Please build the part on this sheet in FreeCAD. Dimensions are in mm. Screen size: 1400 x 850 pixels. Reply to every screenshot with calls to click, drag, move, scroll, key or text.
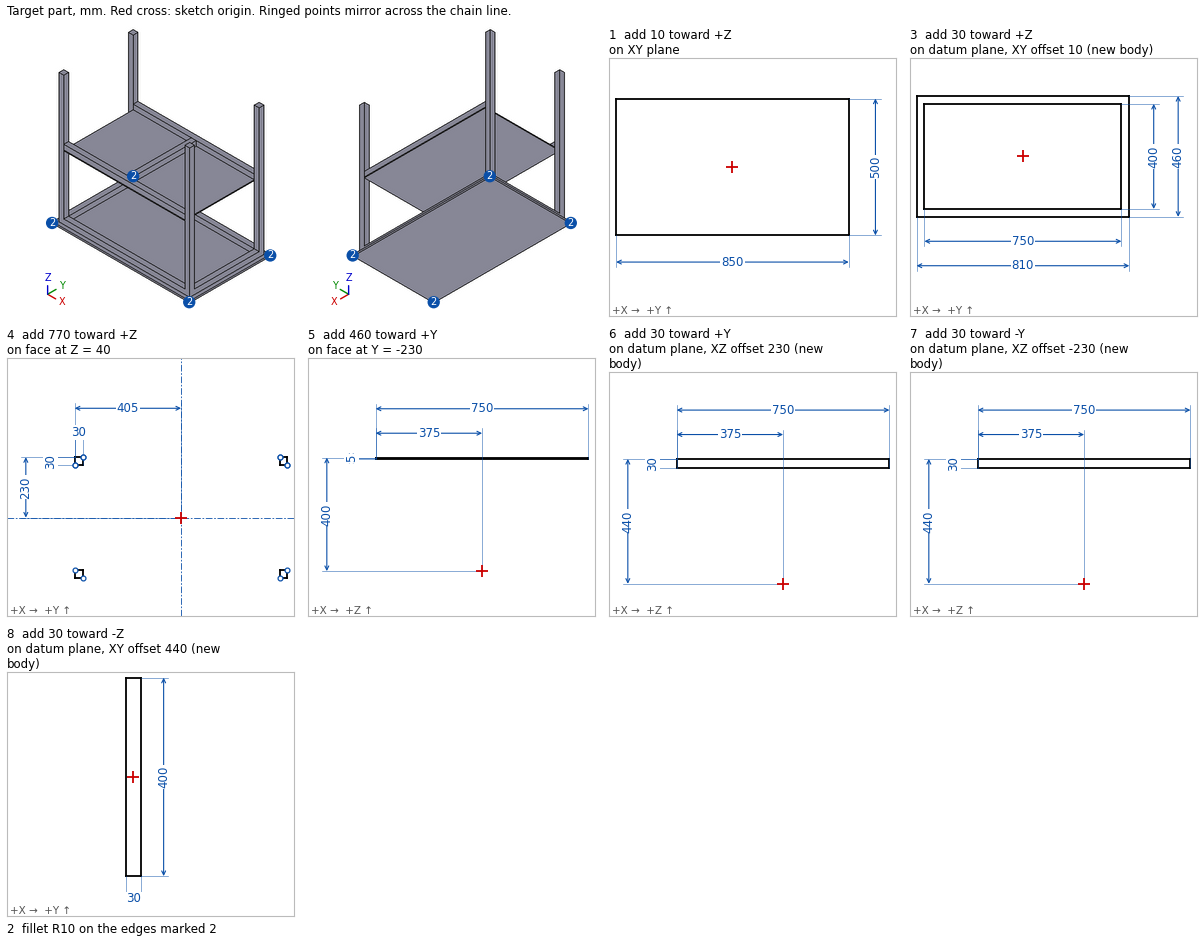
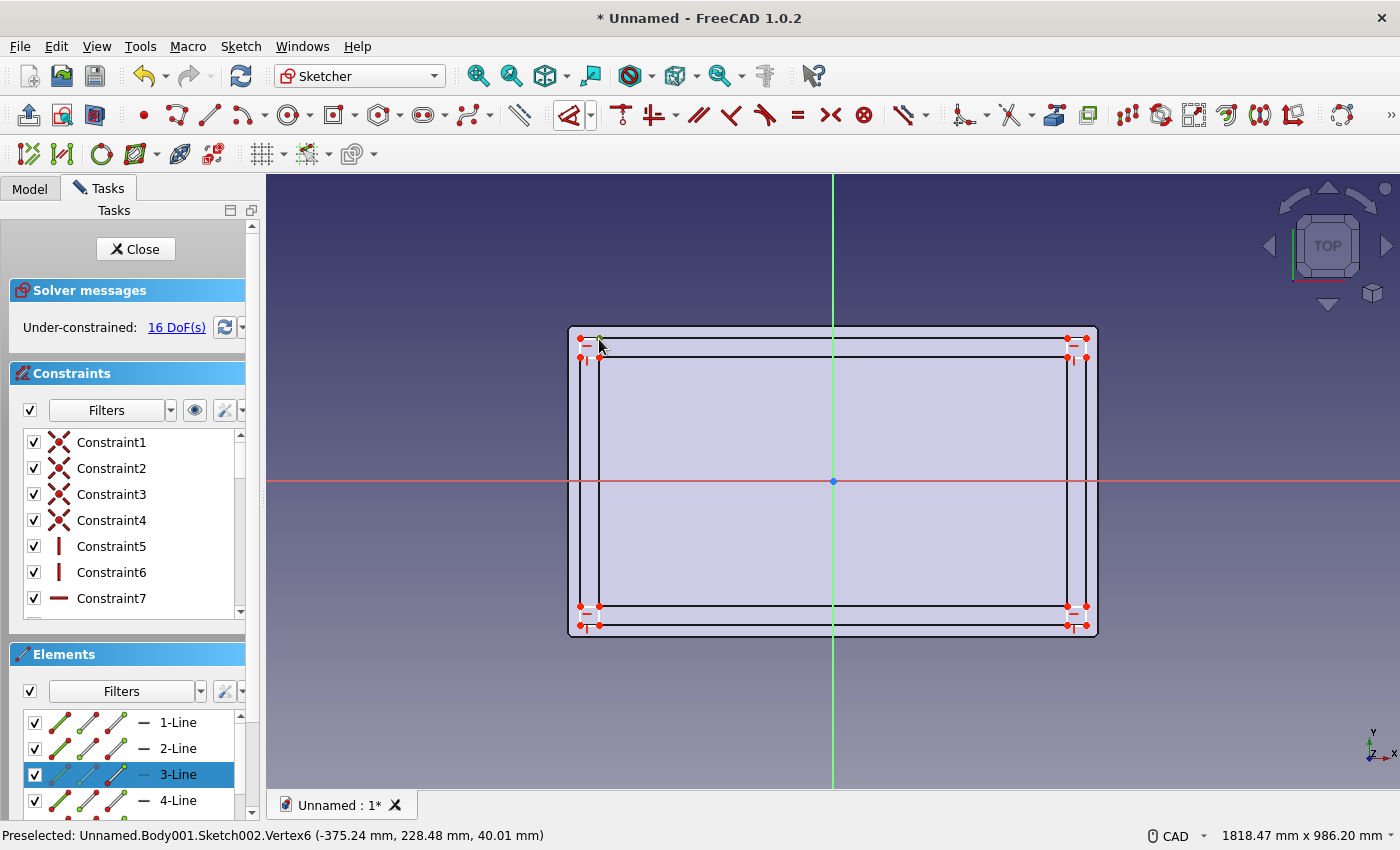
click(1067, 339)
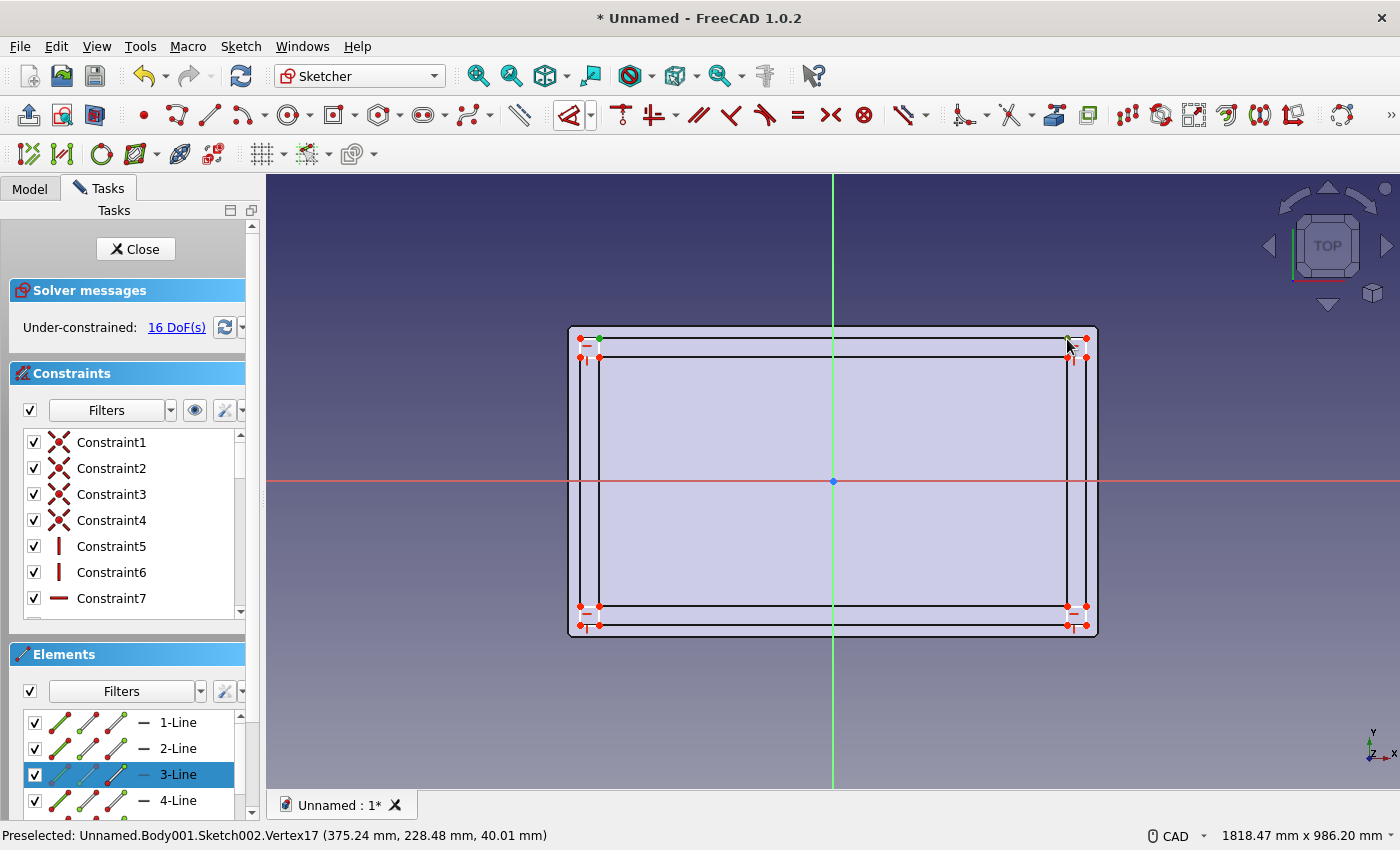
click(833, 721)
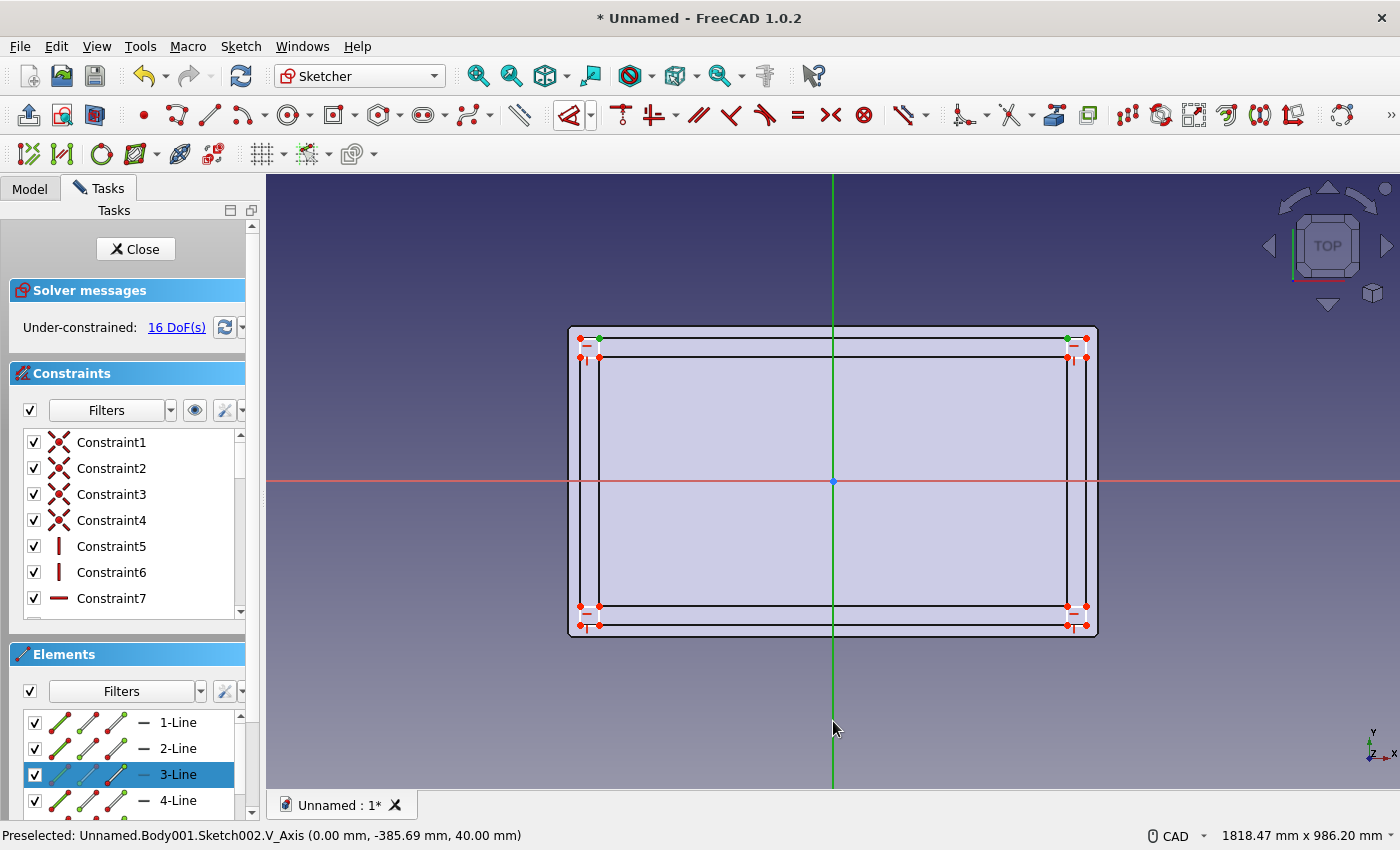
click(831, 116)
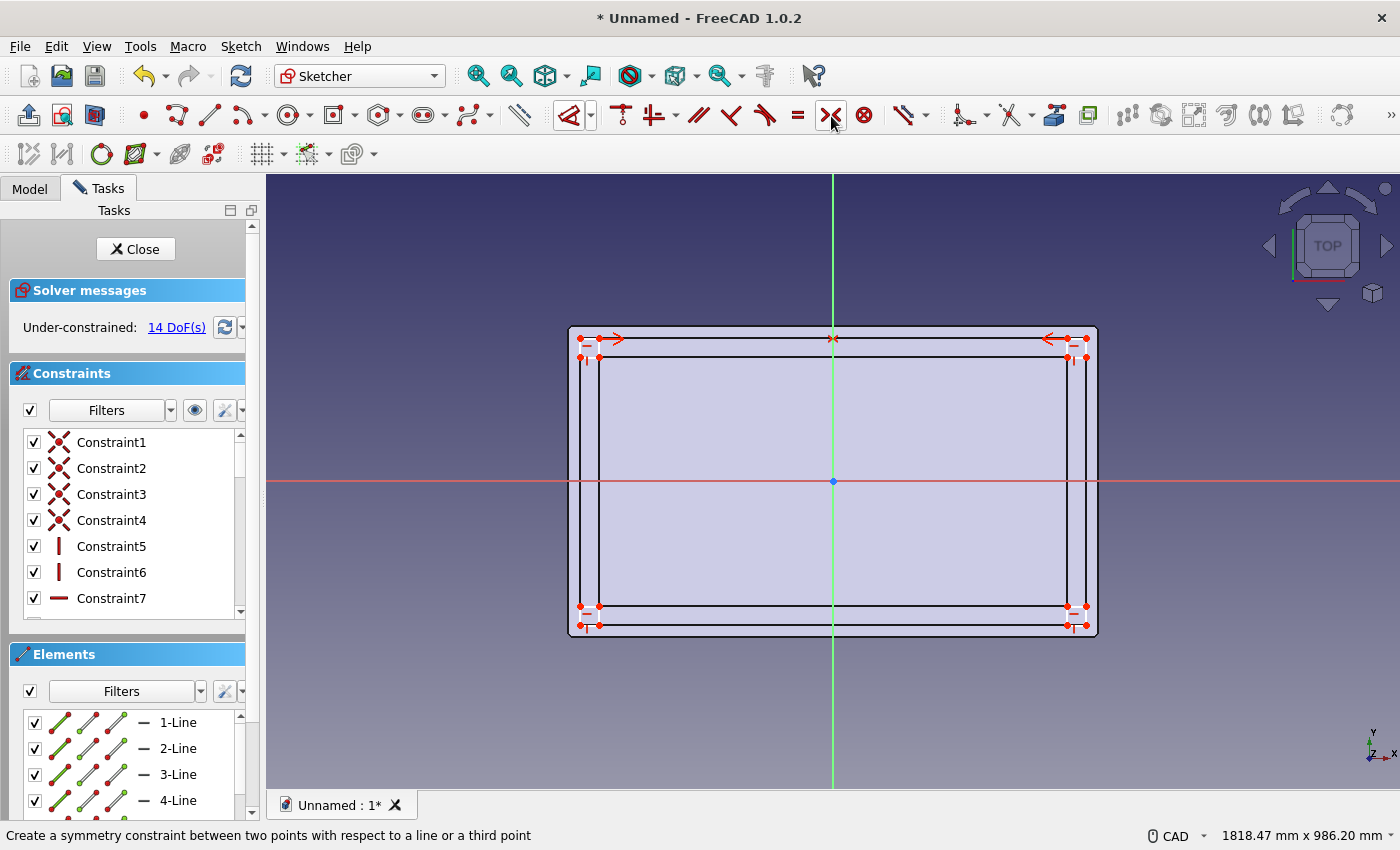
click(1067, 626)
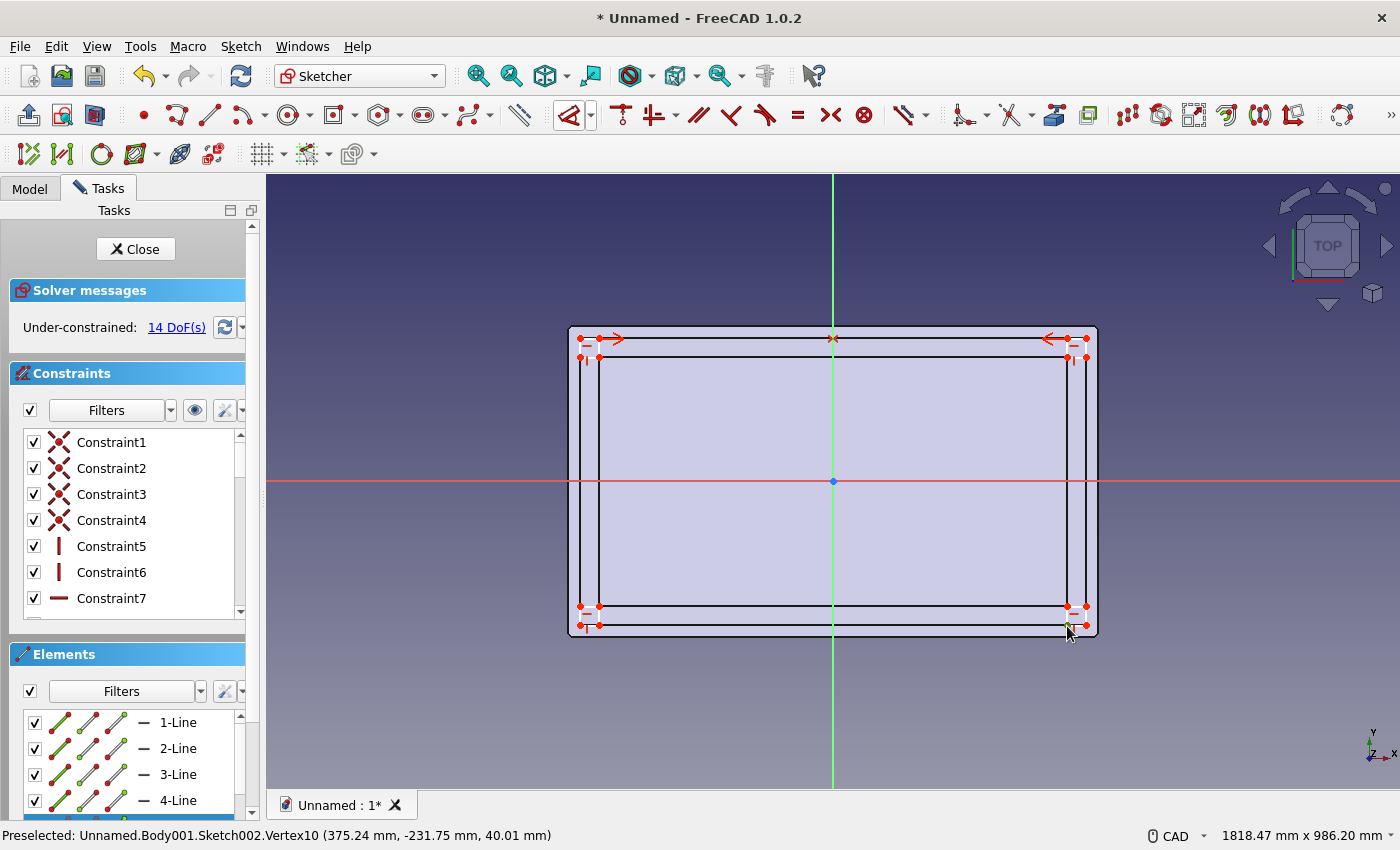
click(1067, 339)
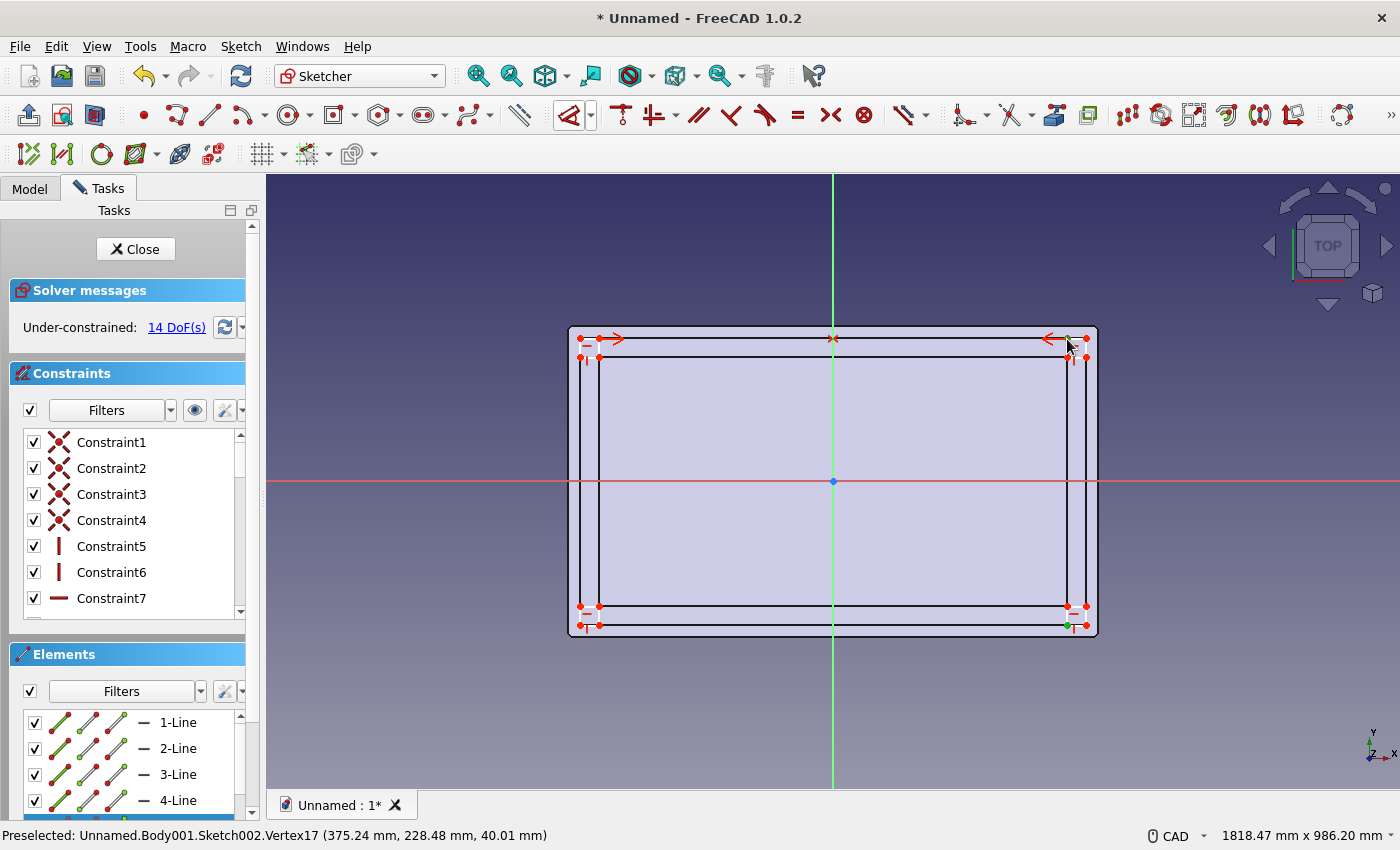
click(361, 481)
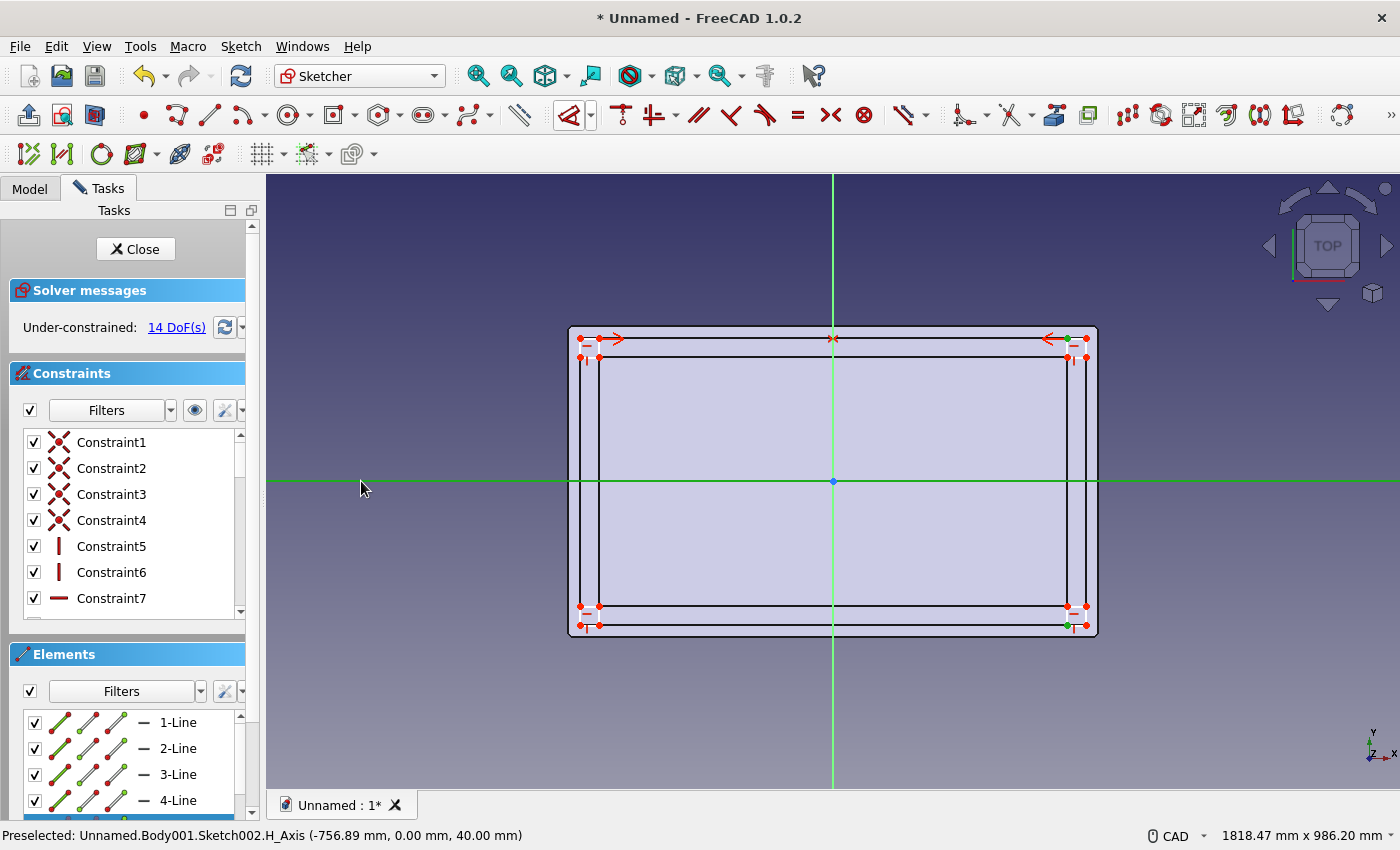
click(831, 116)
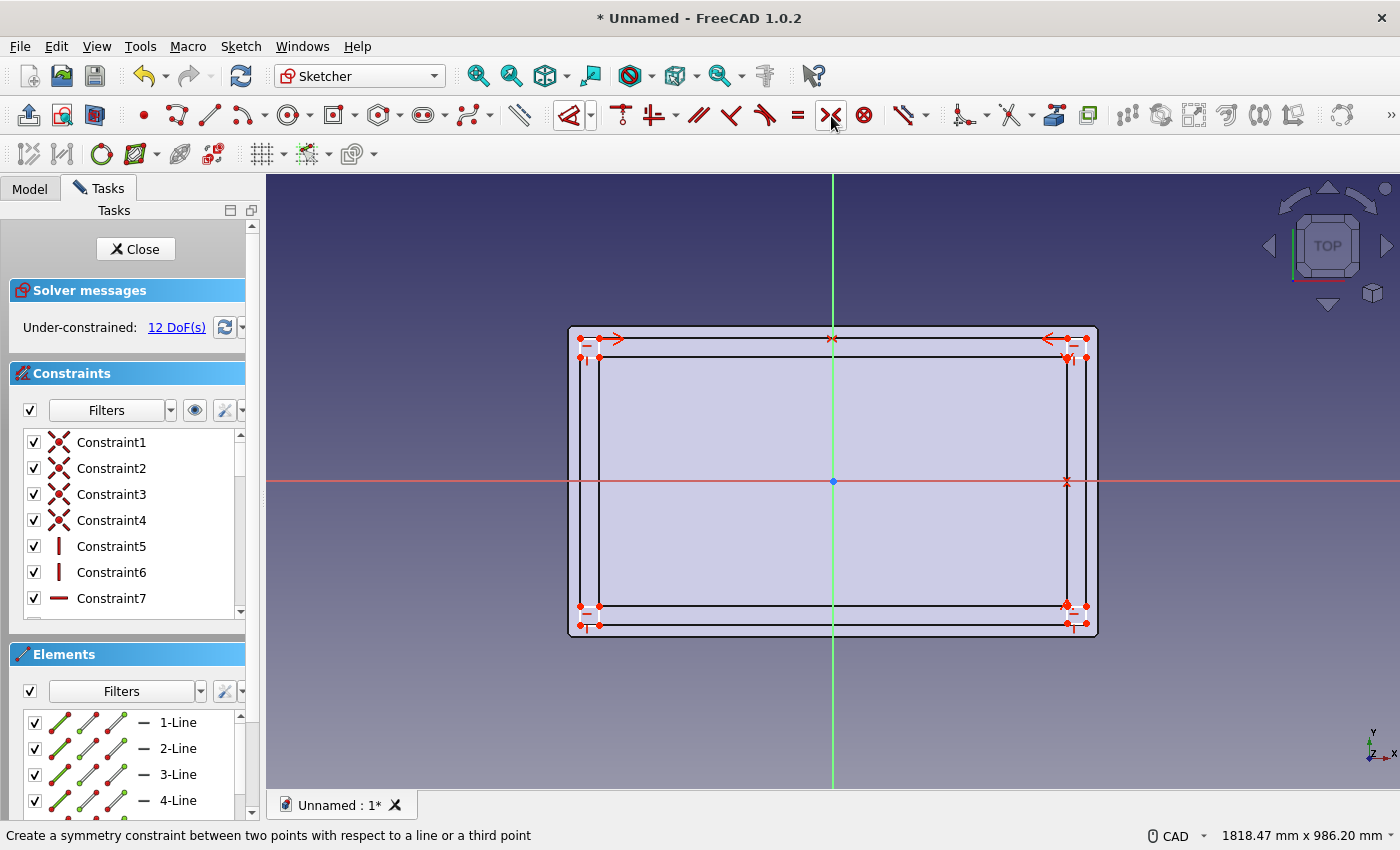
click(580, 358)